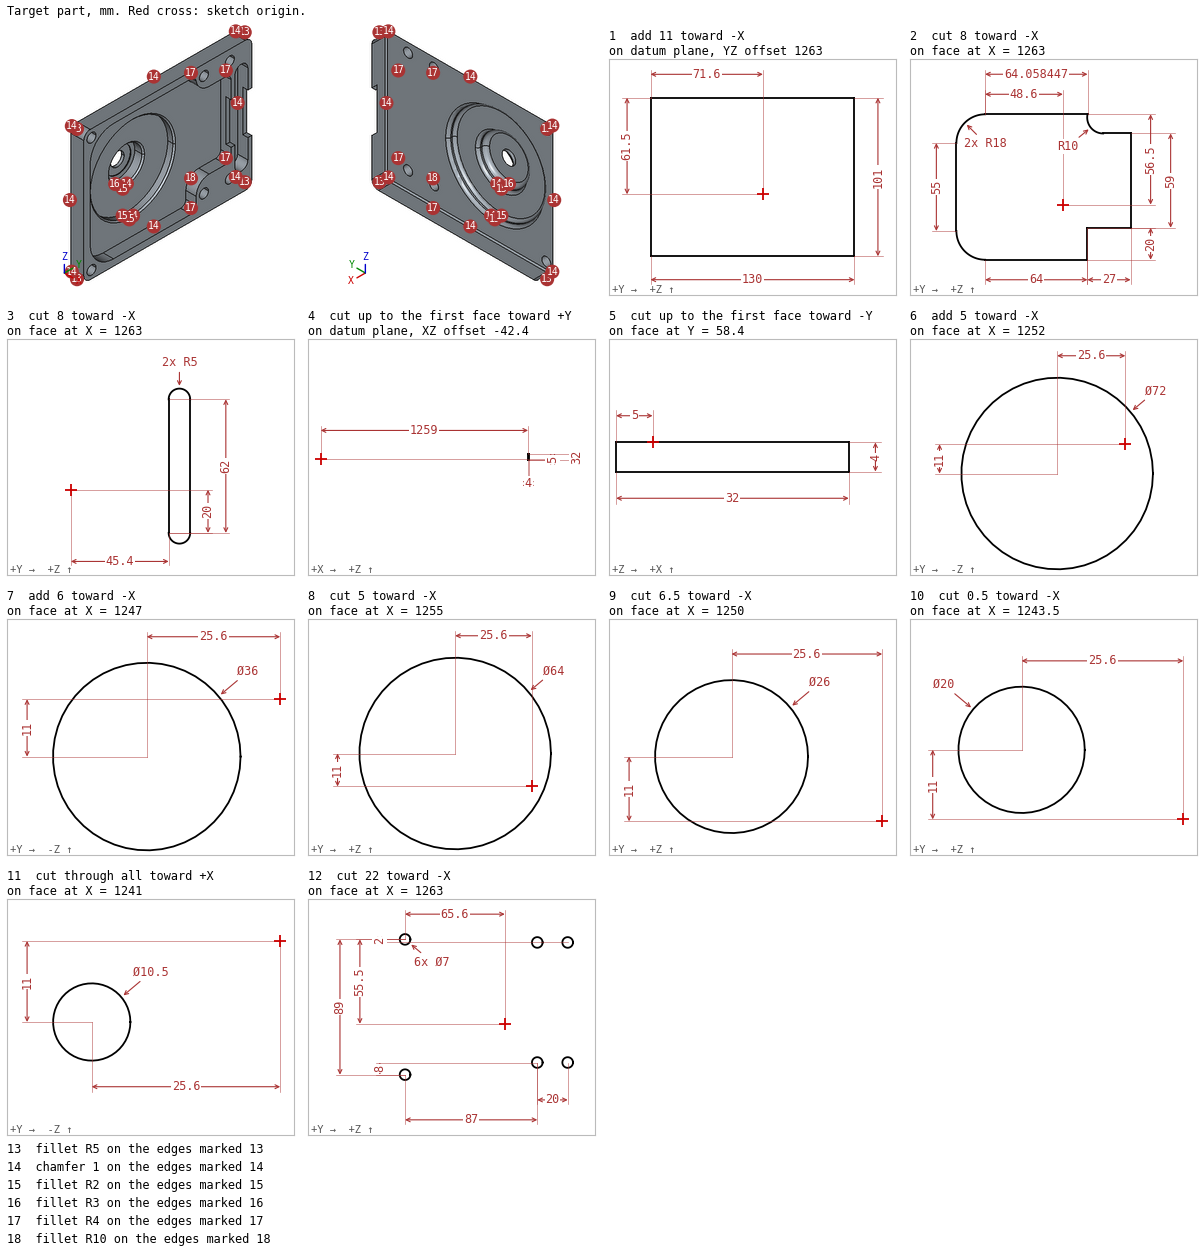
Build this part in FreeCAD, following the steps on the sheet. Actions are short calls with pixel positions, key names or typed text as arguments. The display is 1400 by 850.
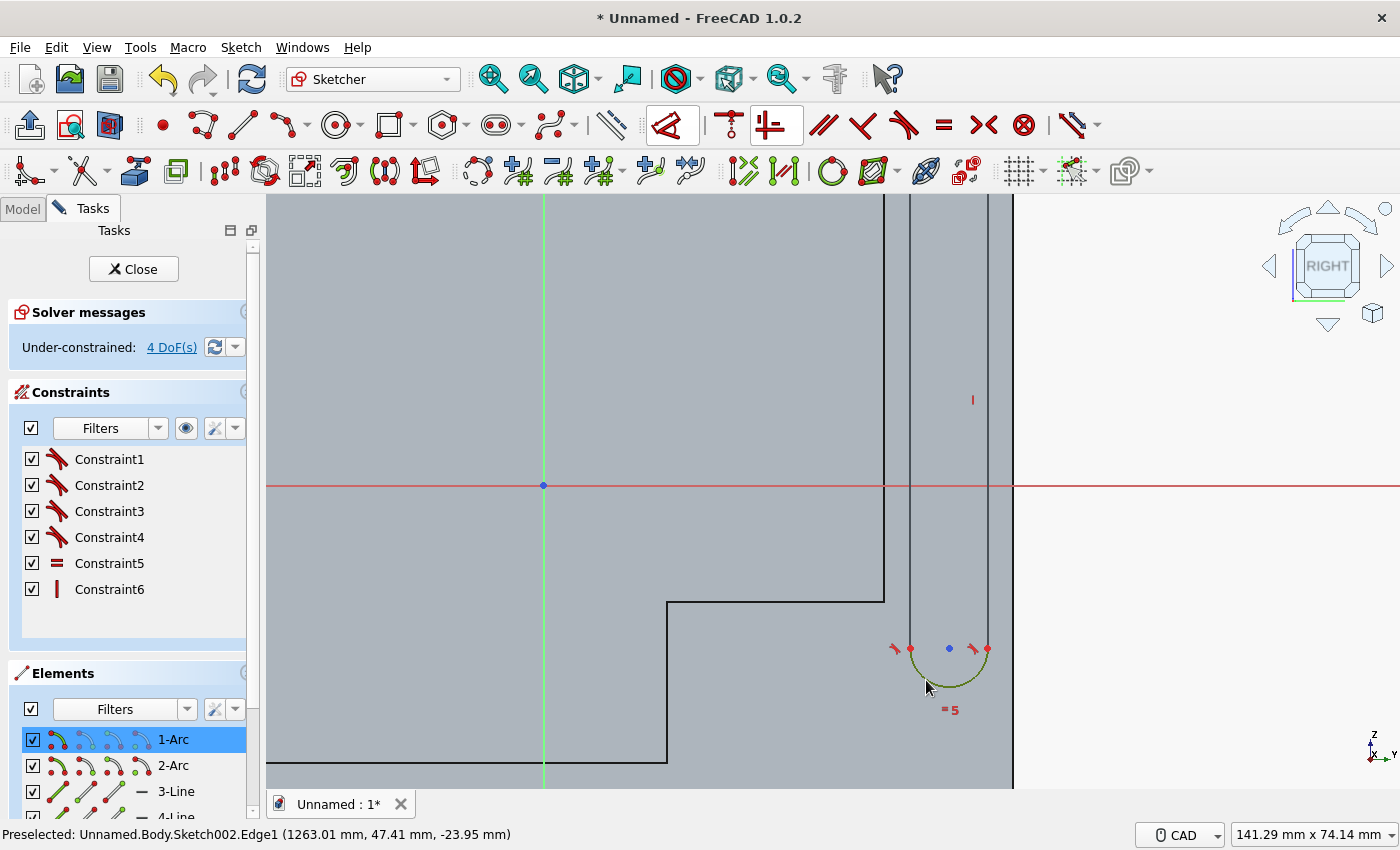
key(k)
key(r)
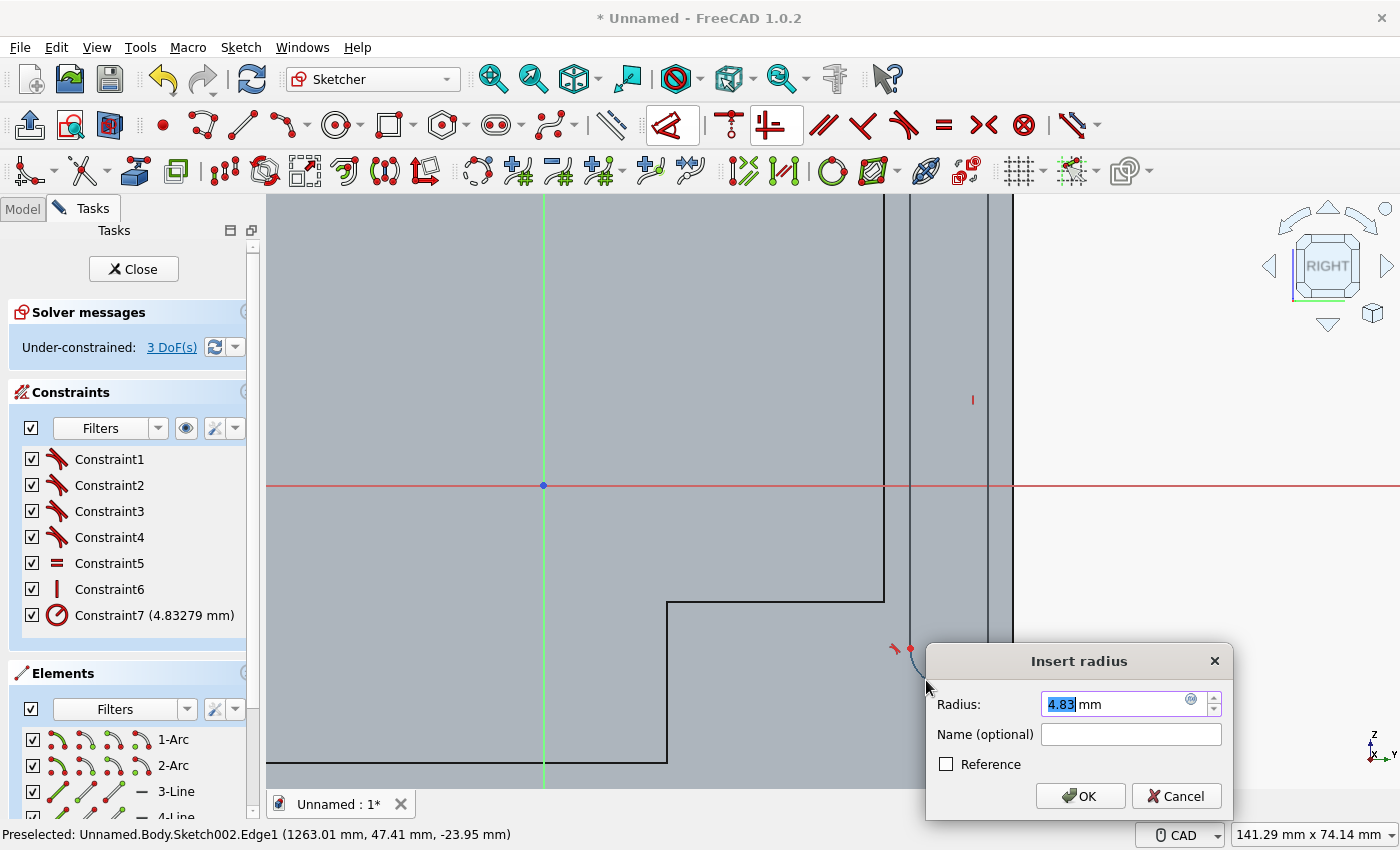
text(5)
key(Return)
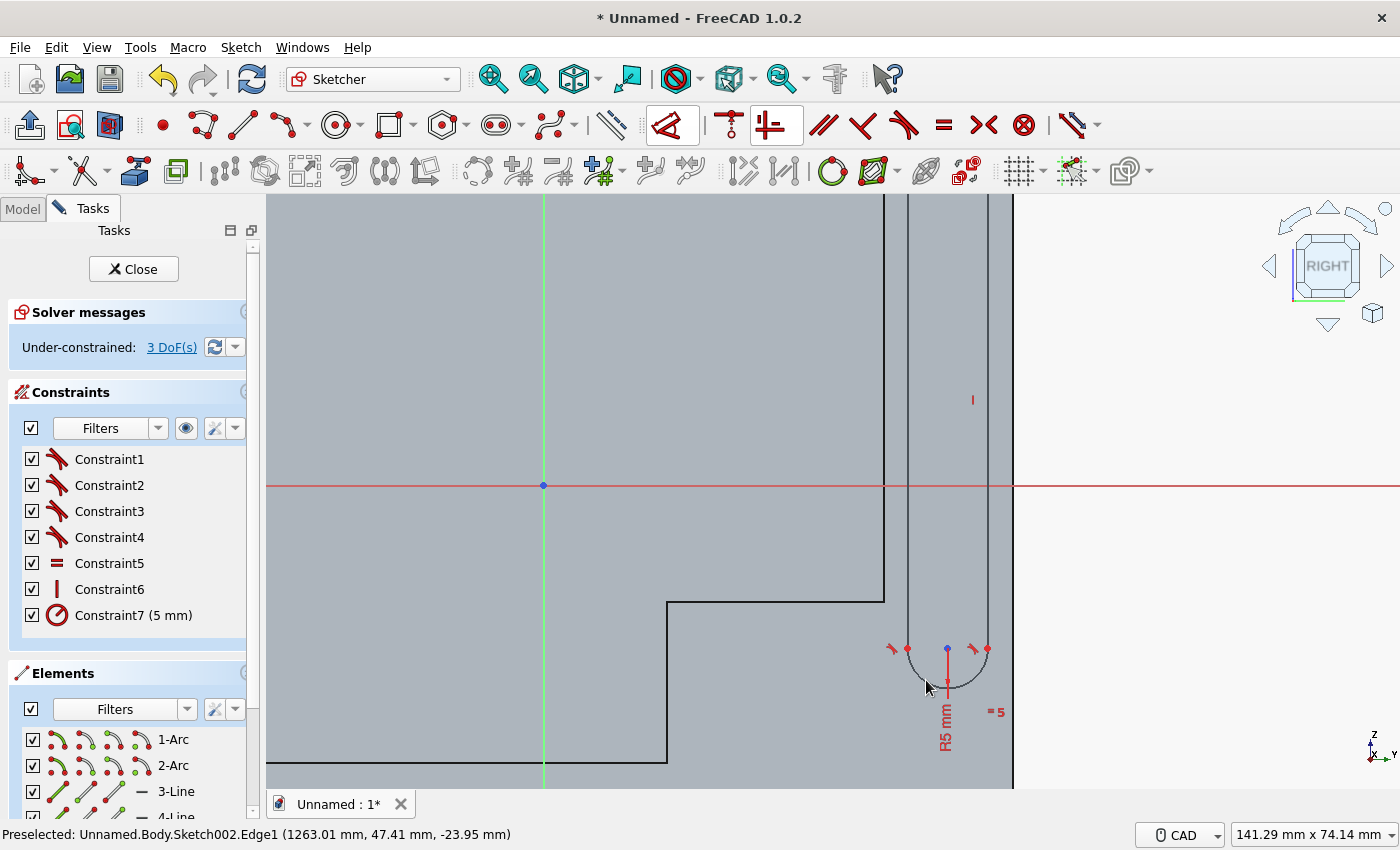
click(908, 499)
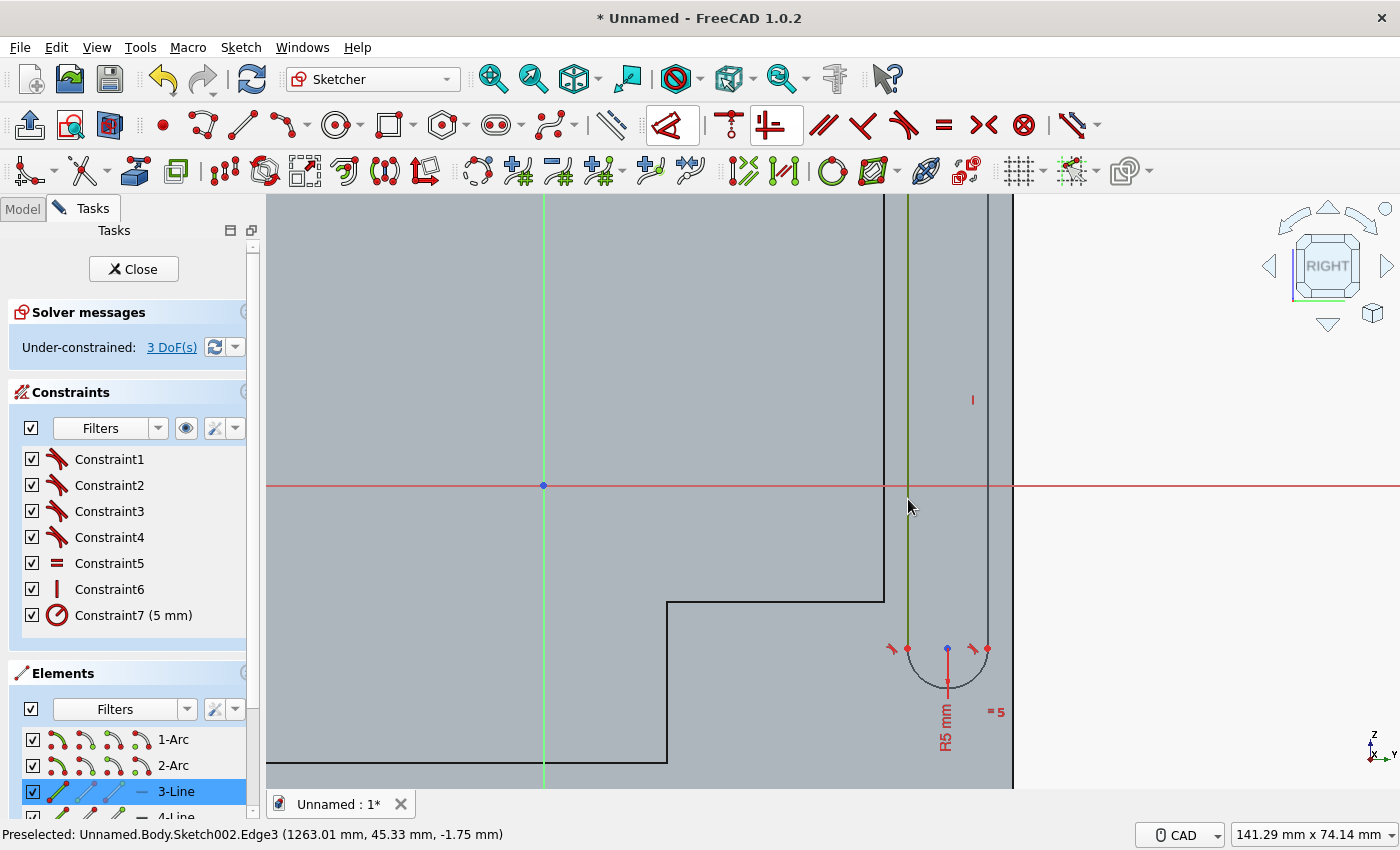
key(i)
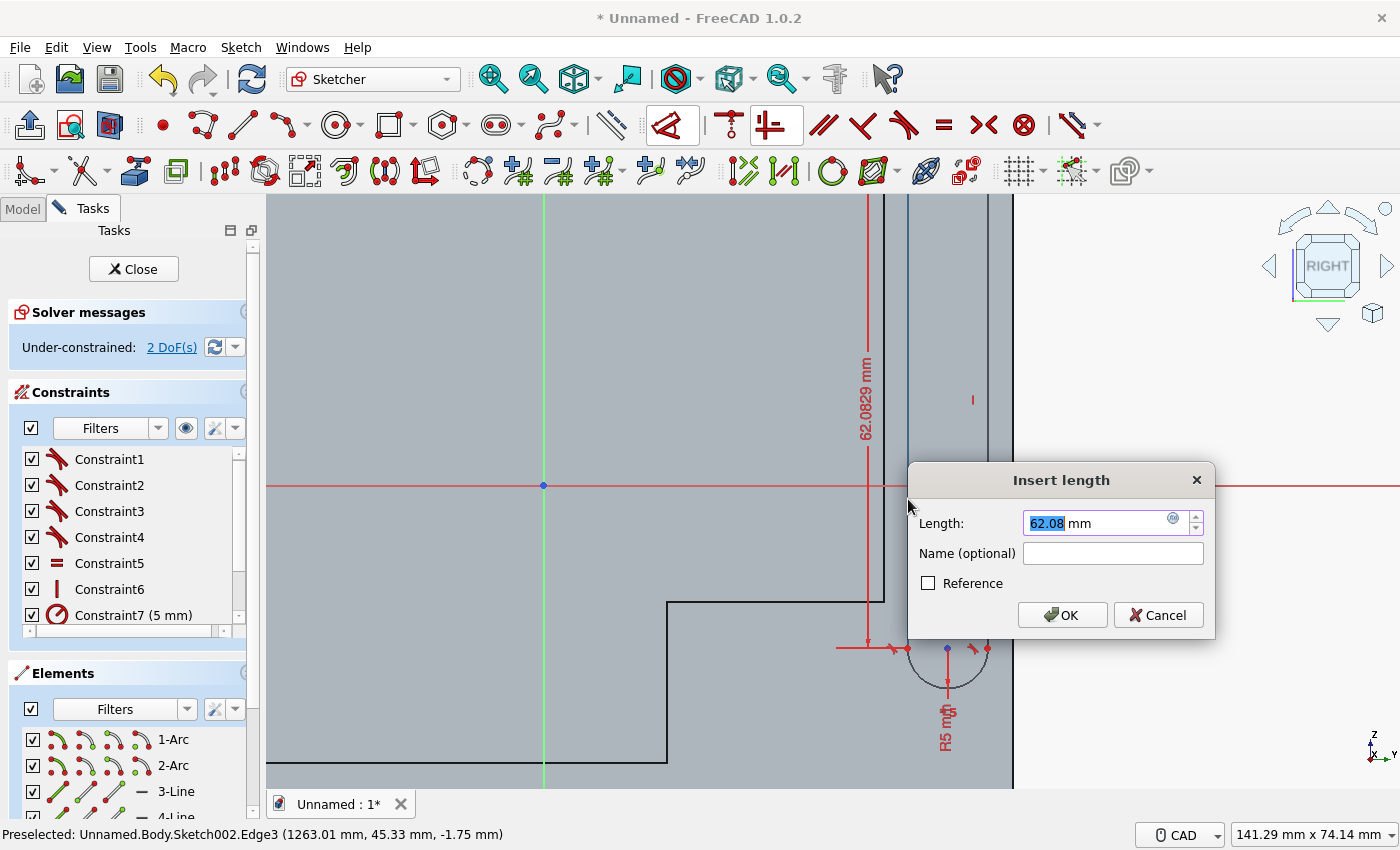
text(62)
key(Return)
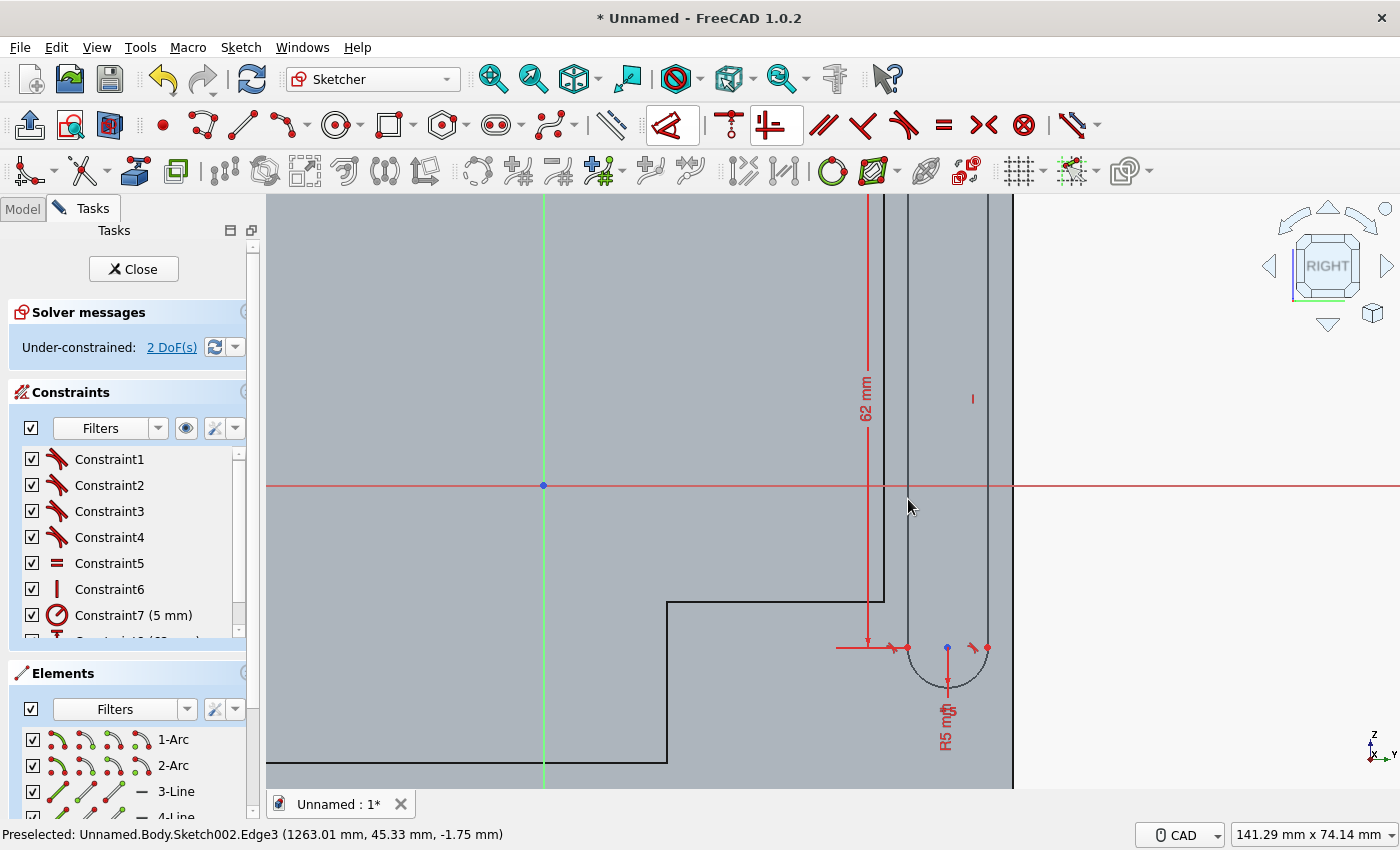
click(908, 648)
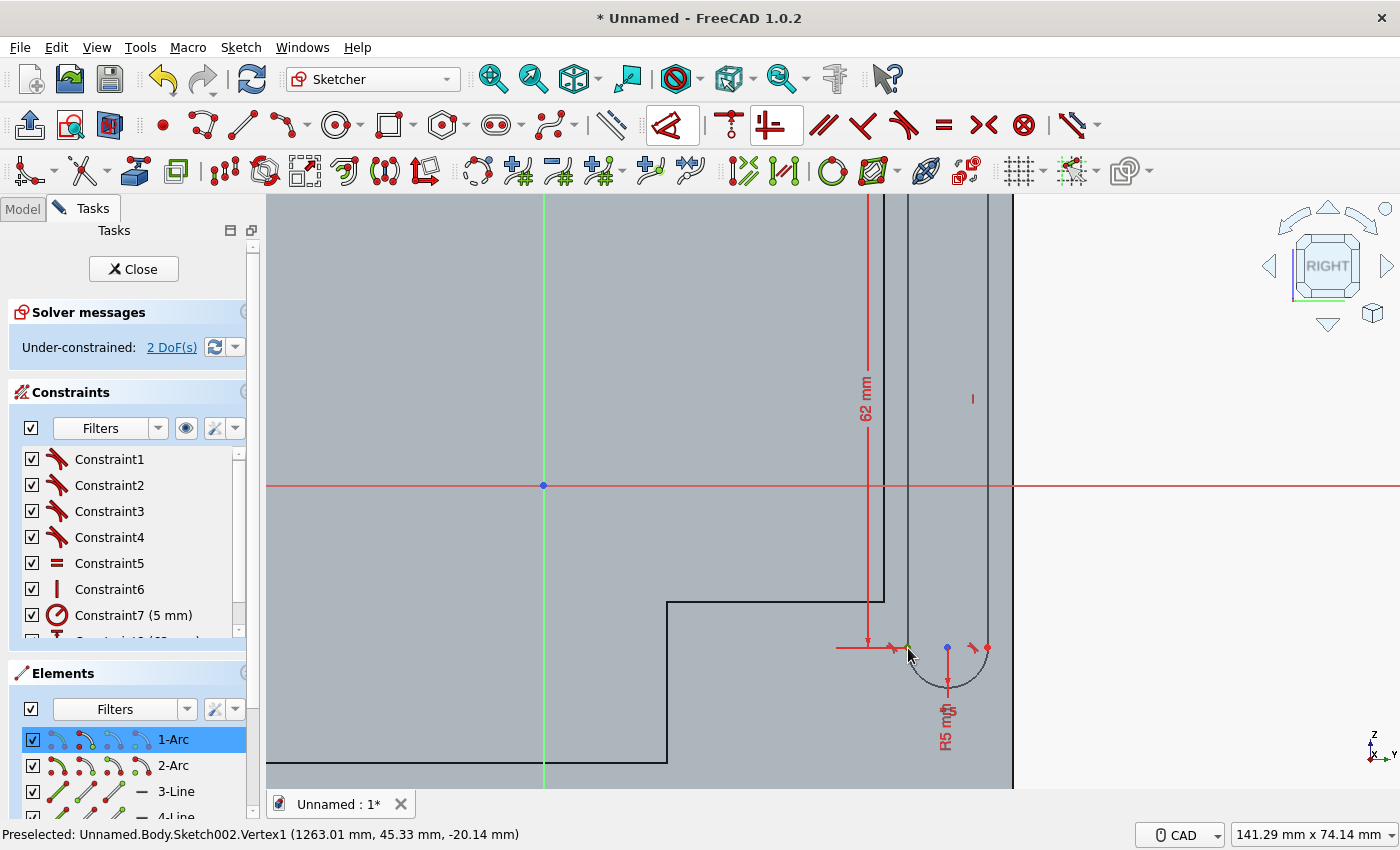
click(694, 126)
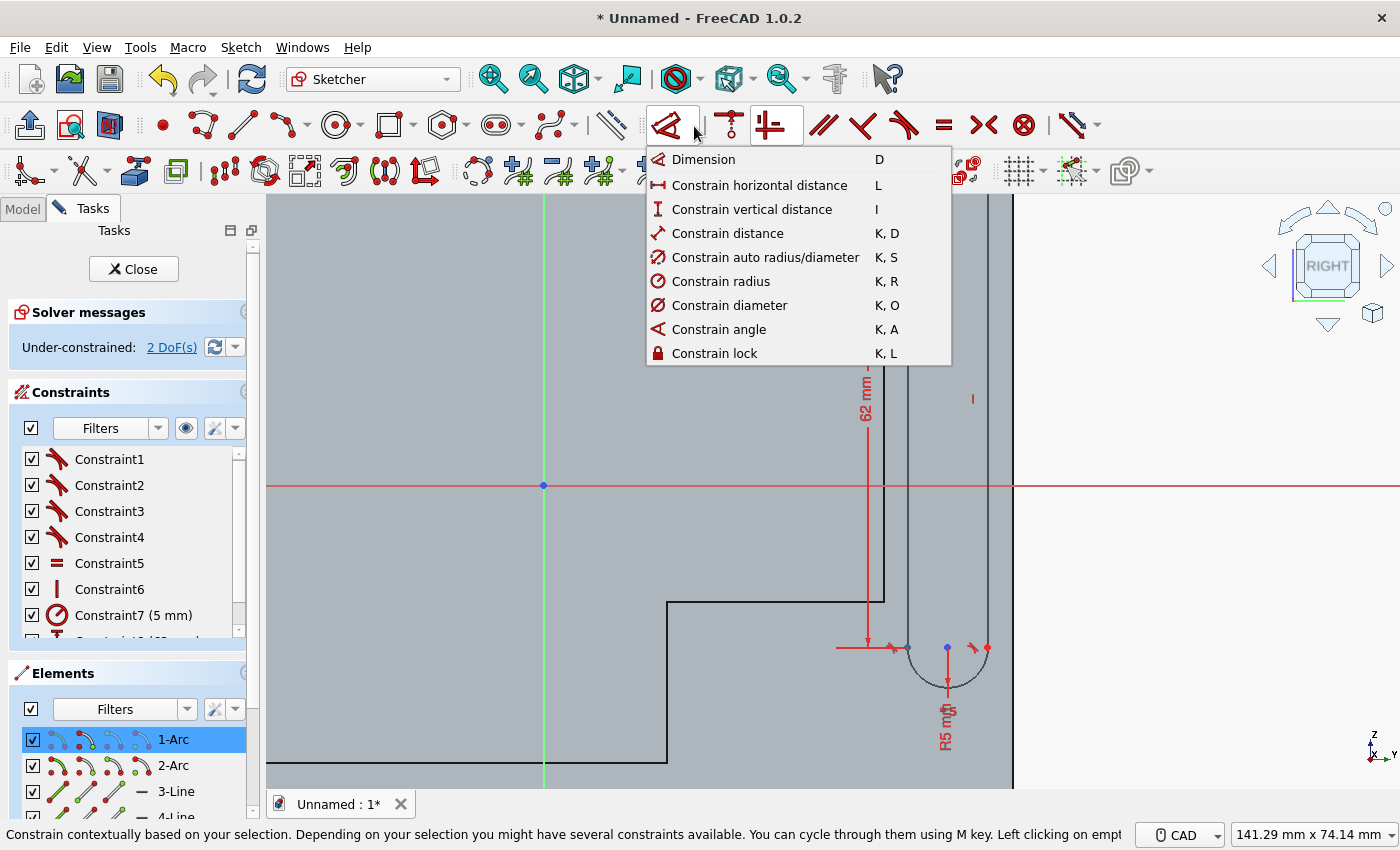
click(799, 209)